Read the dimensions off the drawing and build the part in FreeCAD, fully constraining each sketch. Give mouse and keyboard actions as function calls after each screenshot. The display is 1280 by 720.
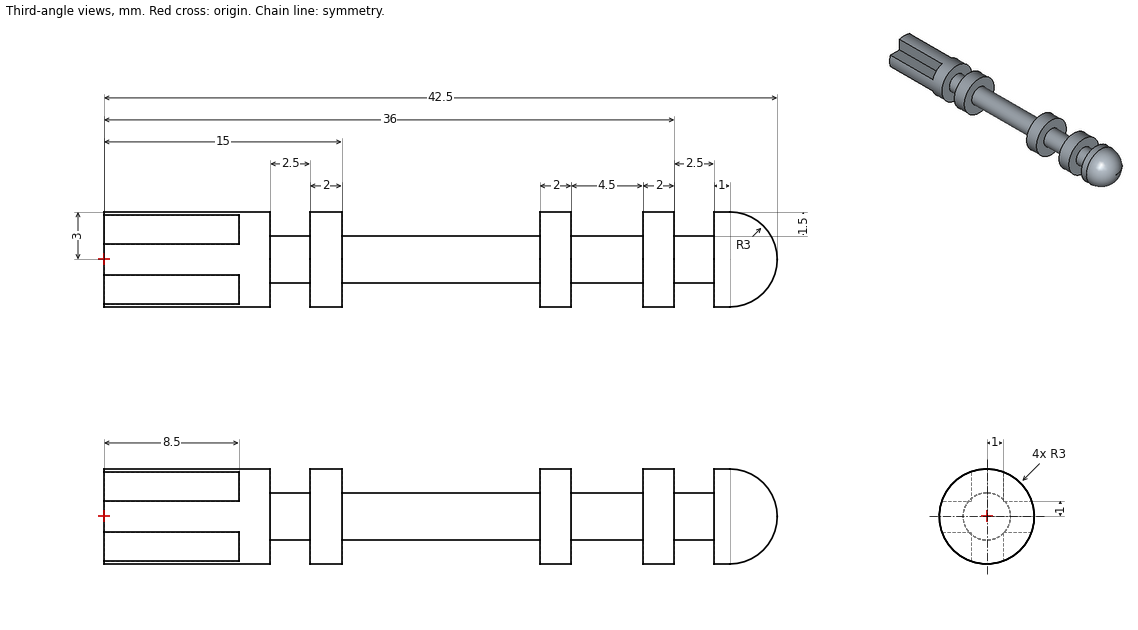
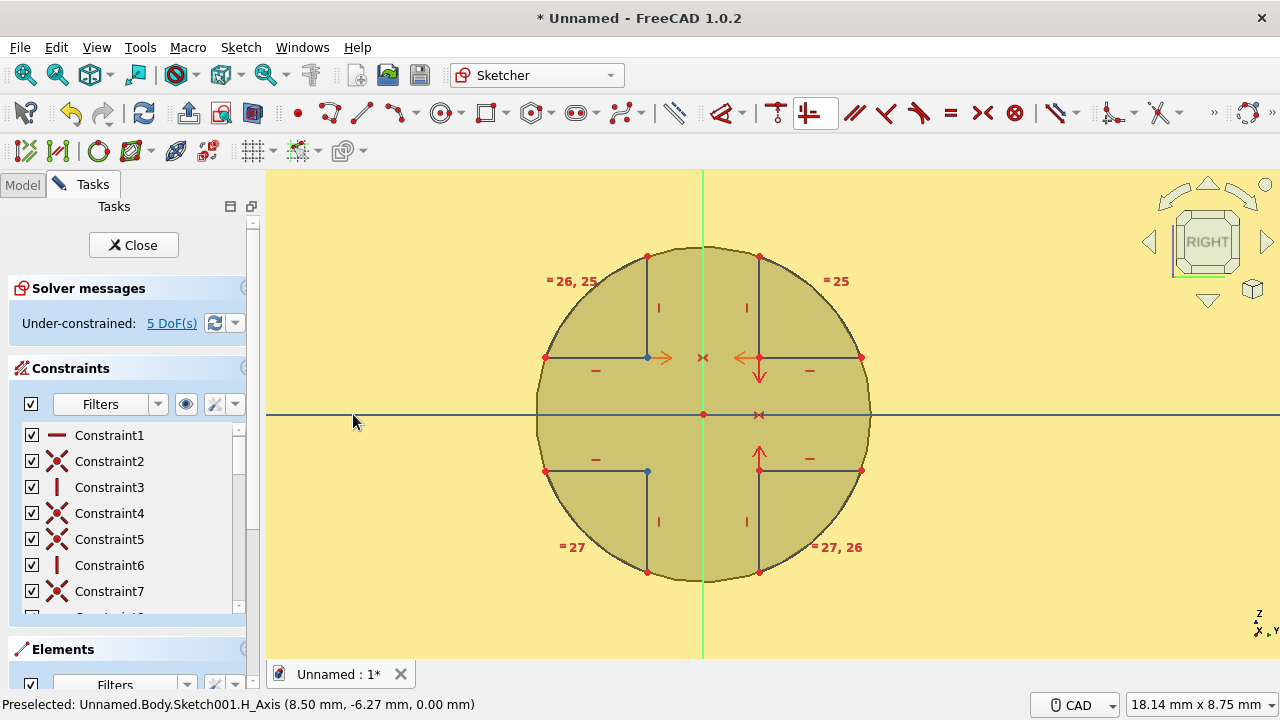
click(984, 114)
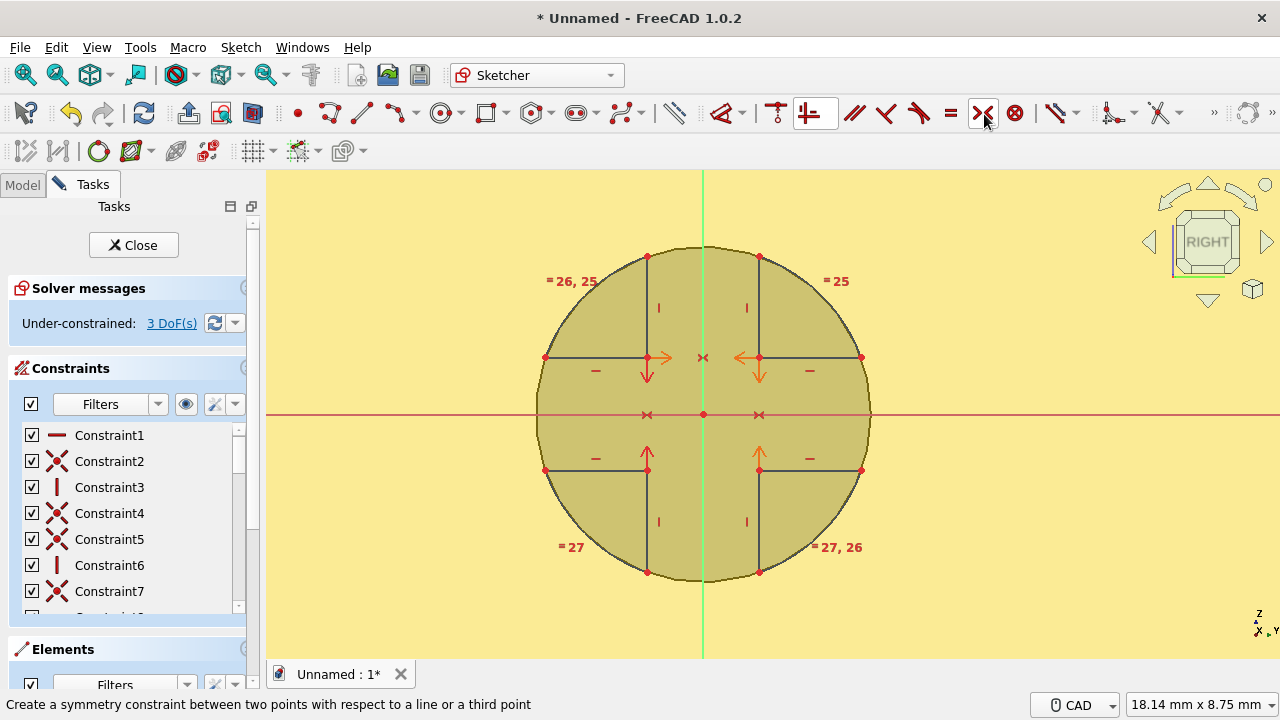
click(722, 114)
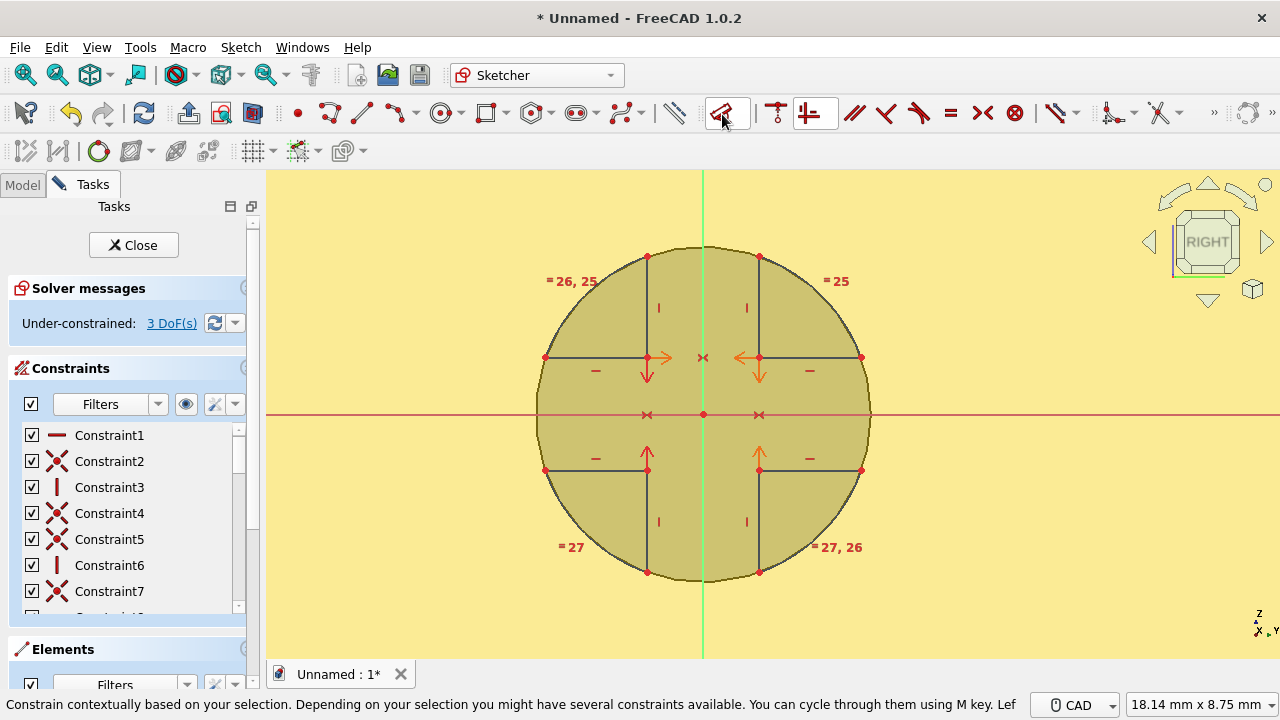
click(841, 319)
click(867, 301)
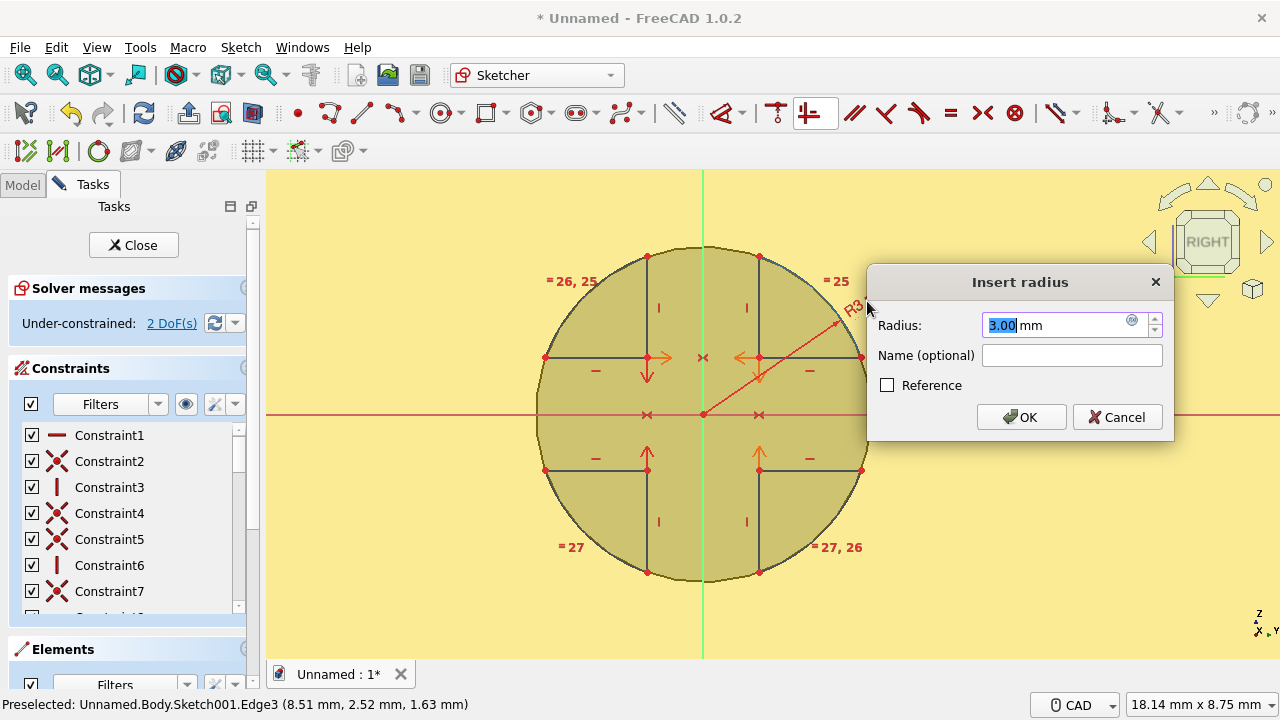
text(3)
key(Return)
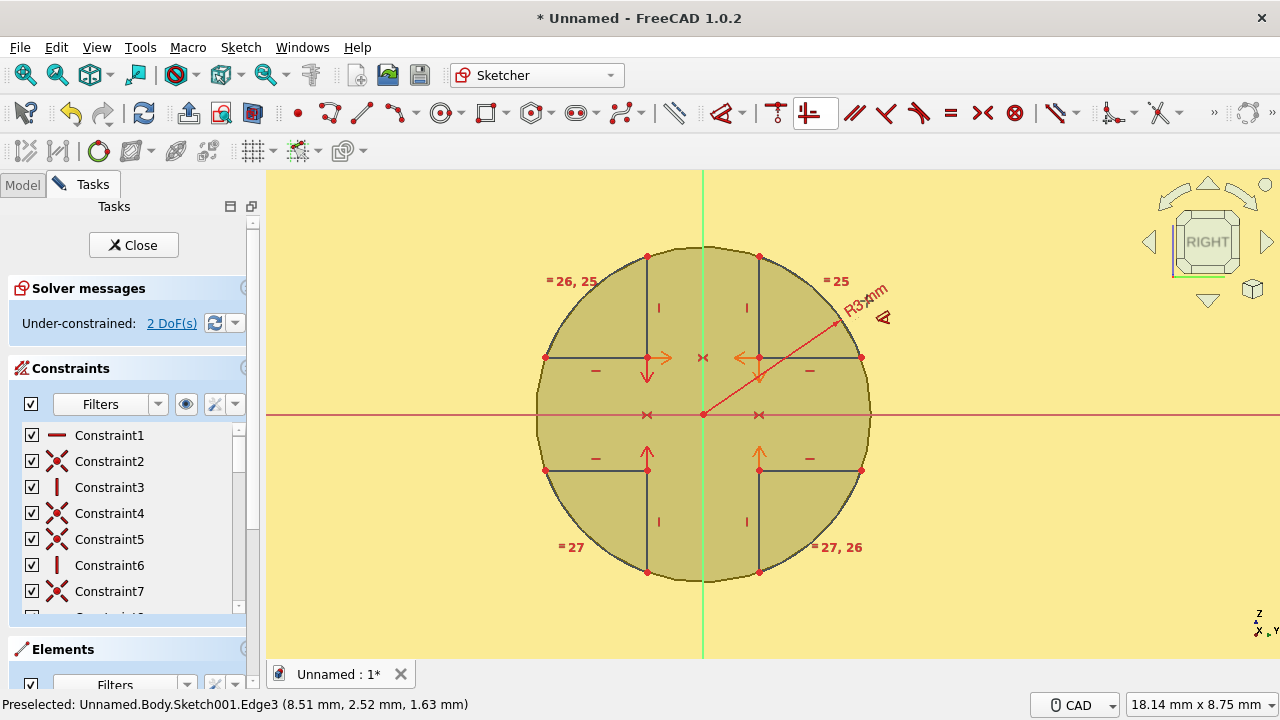
click(861, 358)
click(895, 386)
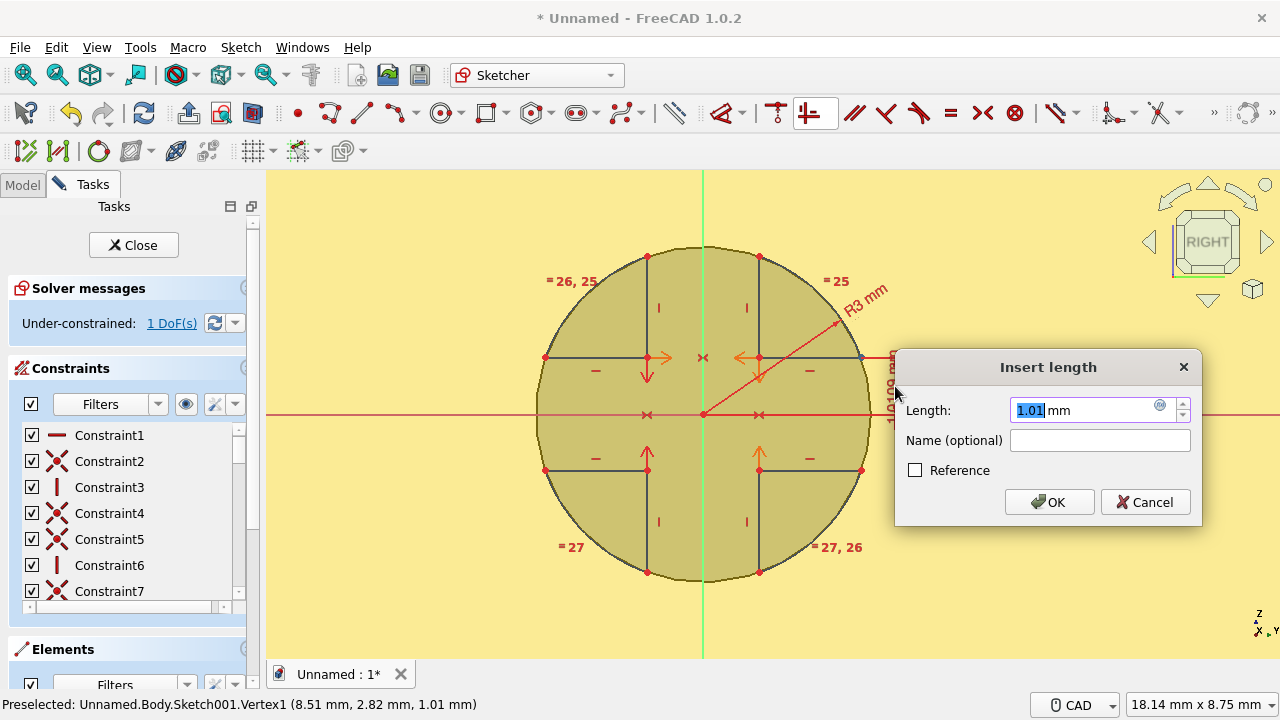
text(1)
key(Return)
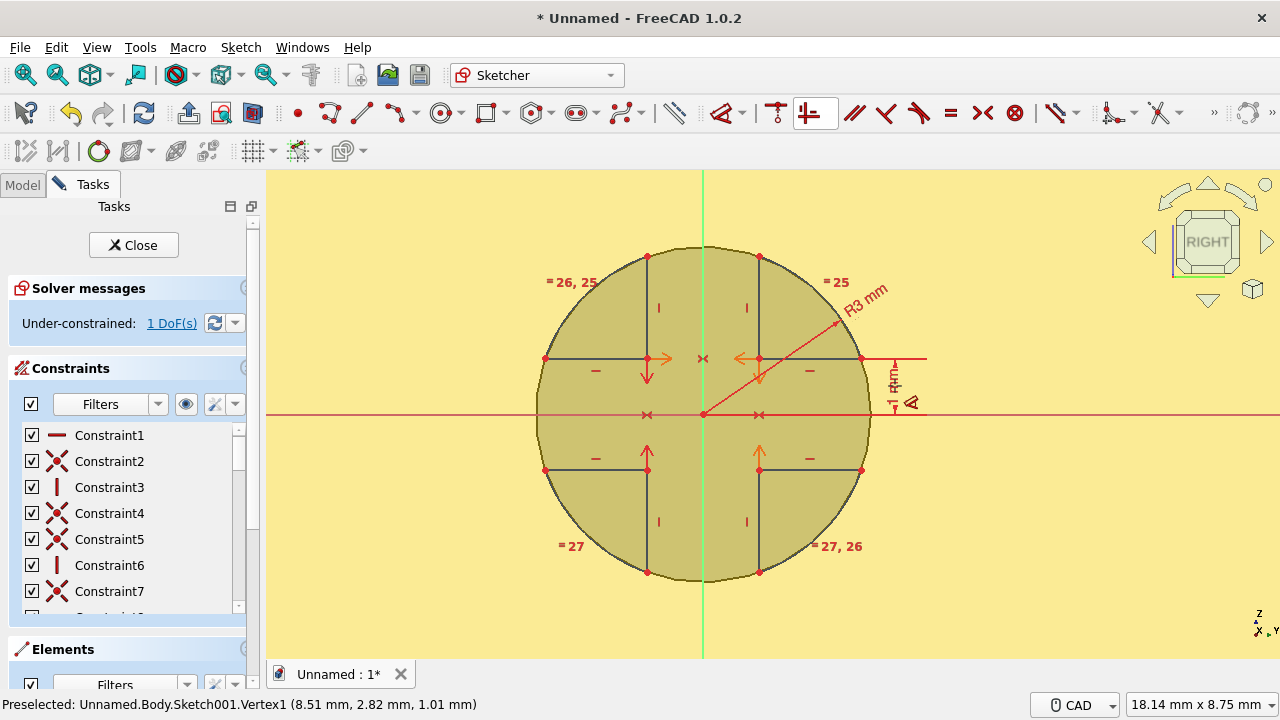
click(759, 359)
click(731, 325)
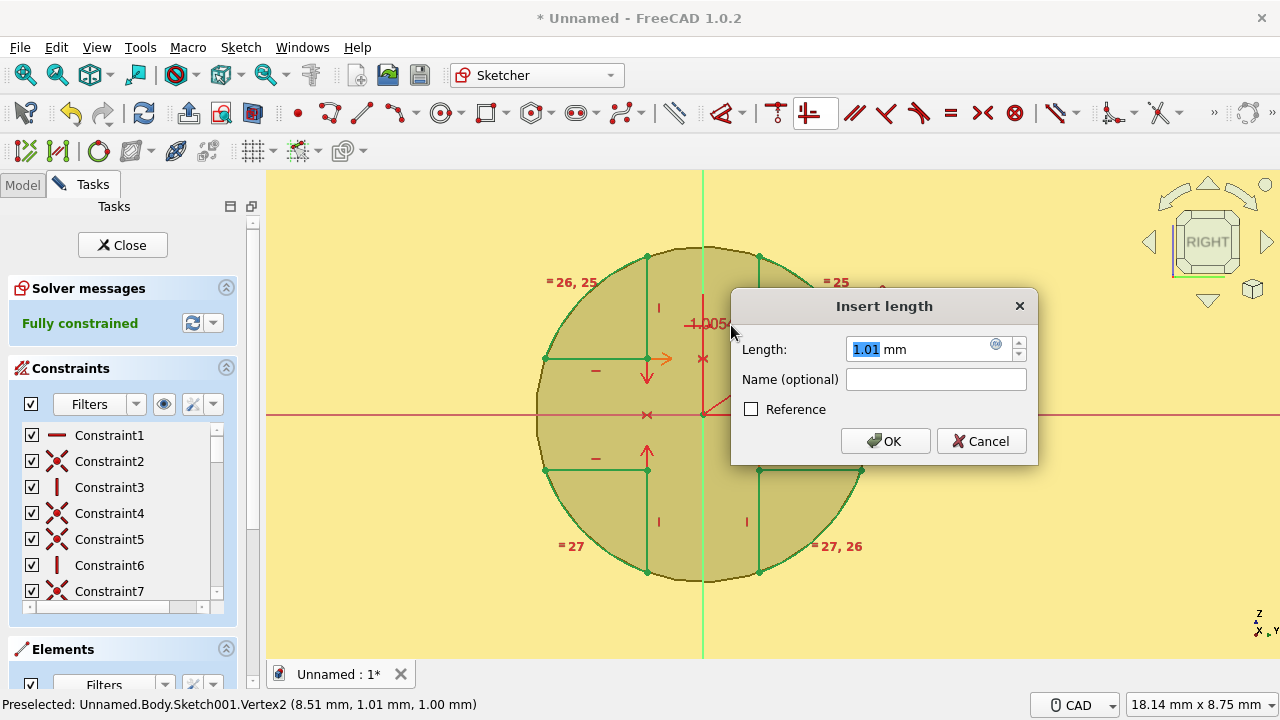
text(1)
key(Return)
key(Escape)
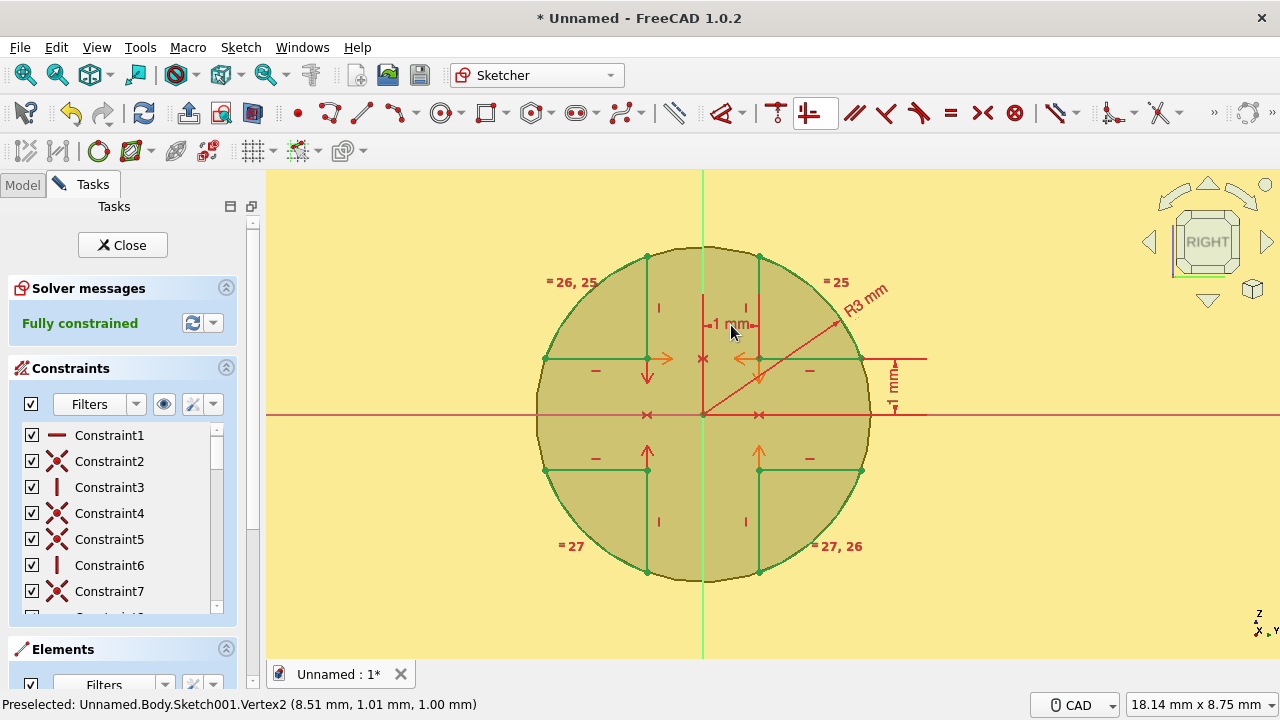
click(123, 245)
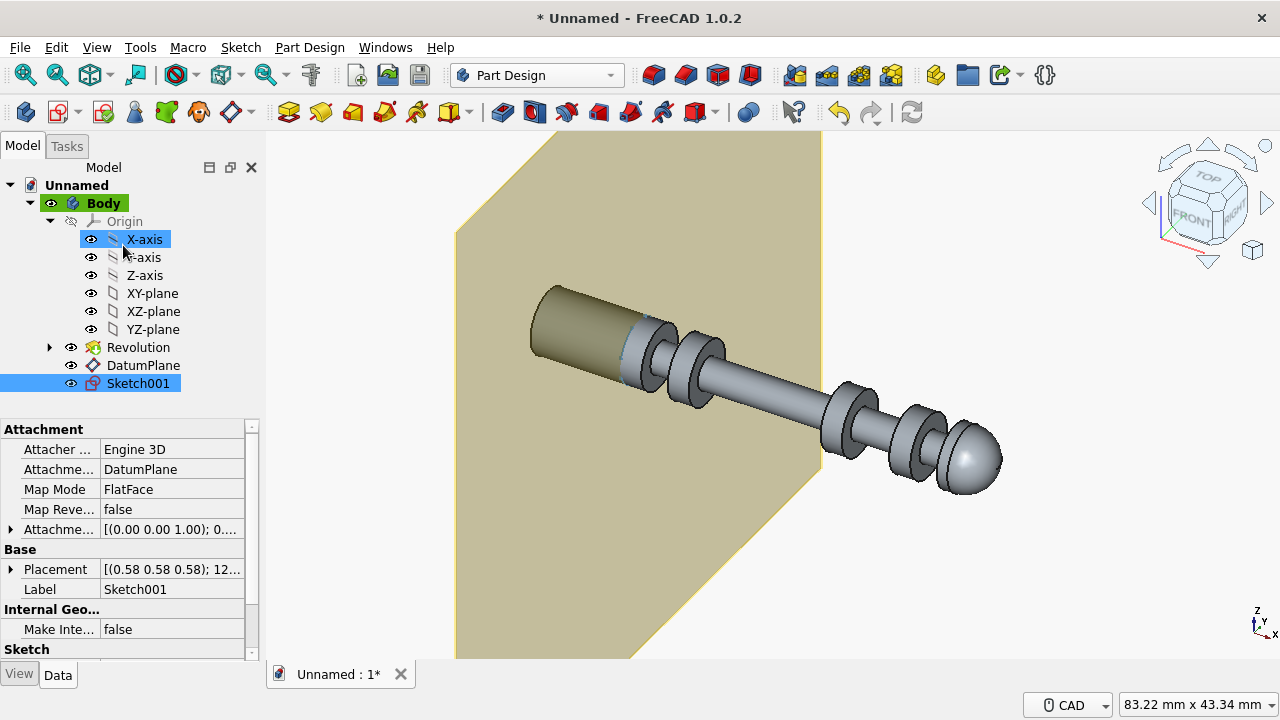
click(504, 112)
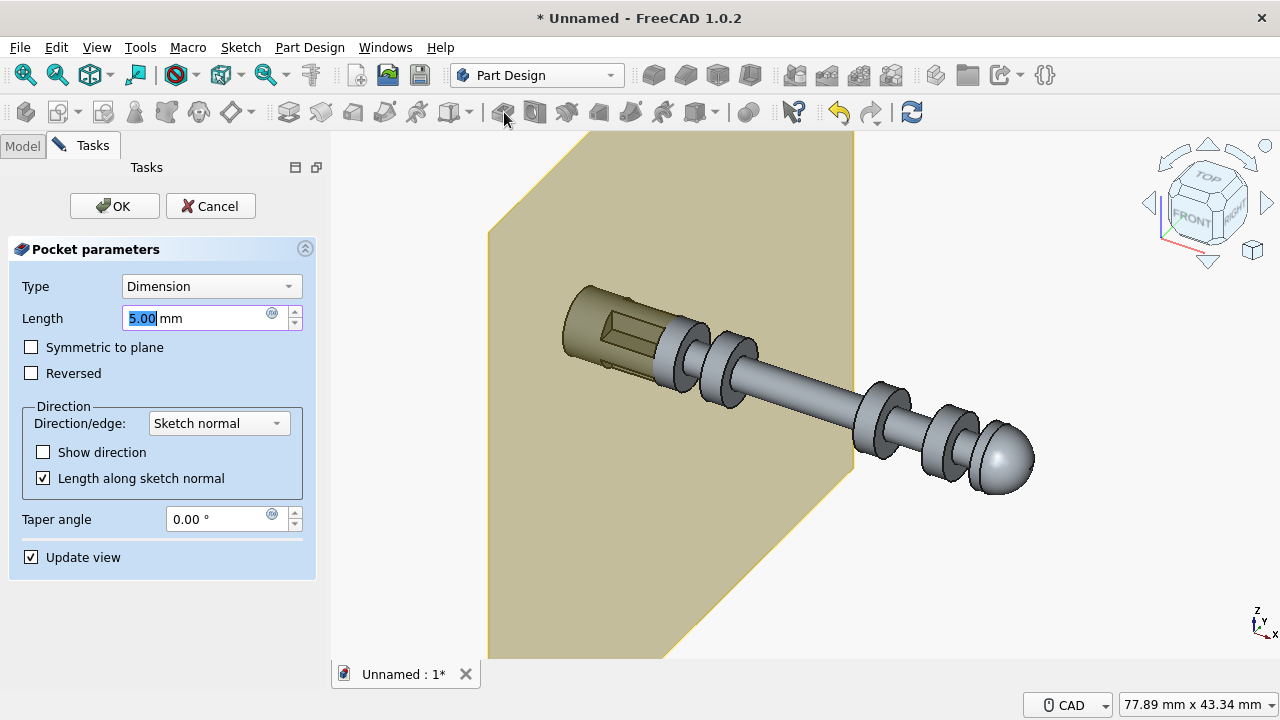
text(8.5)
key(Tab)